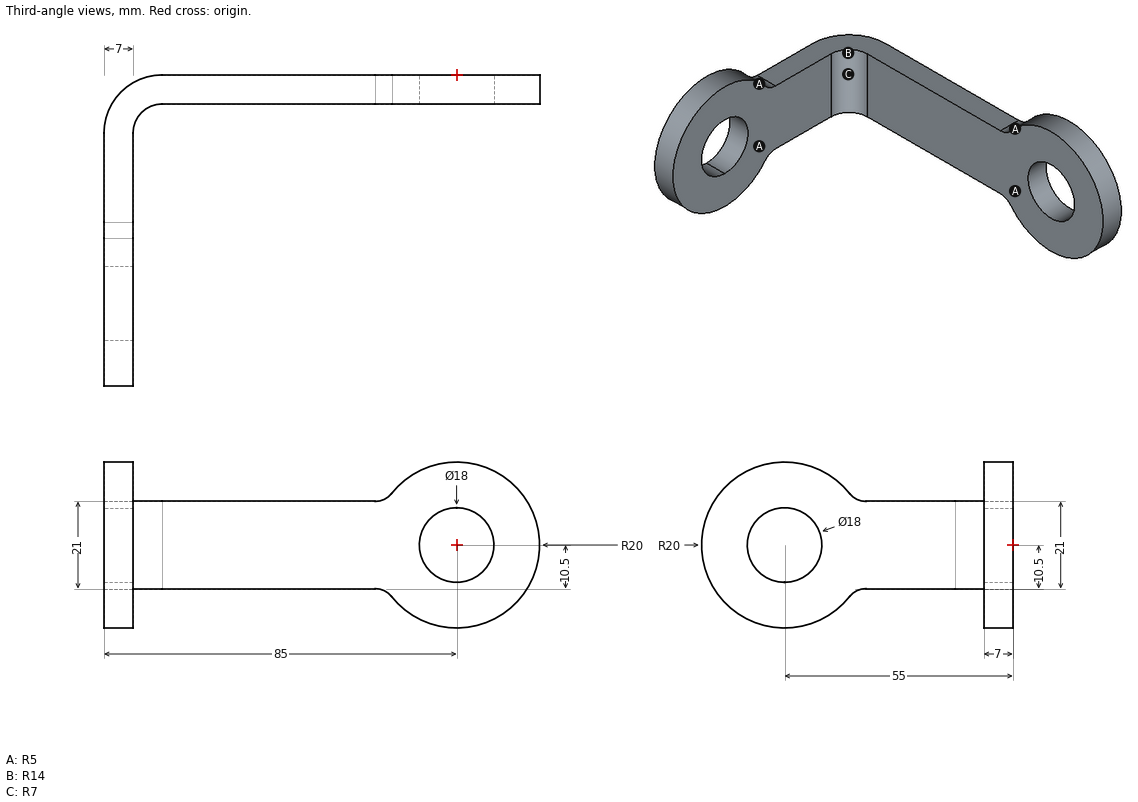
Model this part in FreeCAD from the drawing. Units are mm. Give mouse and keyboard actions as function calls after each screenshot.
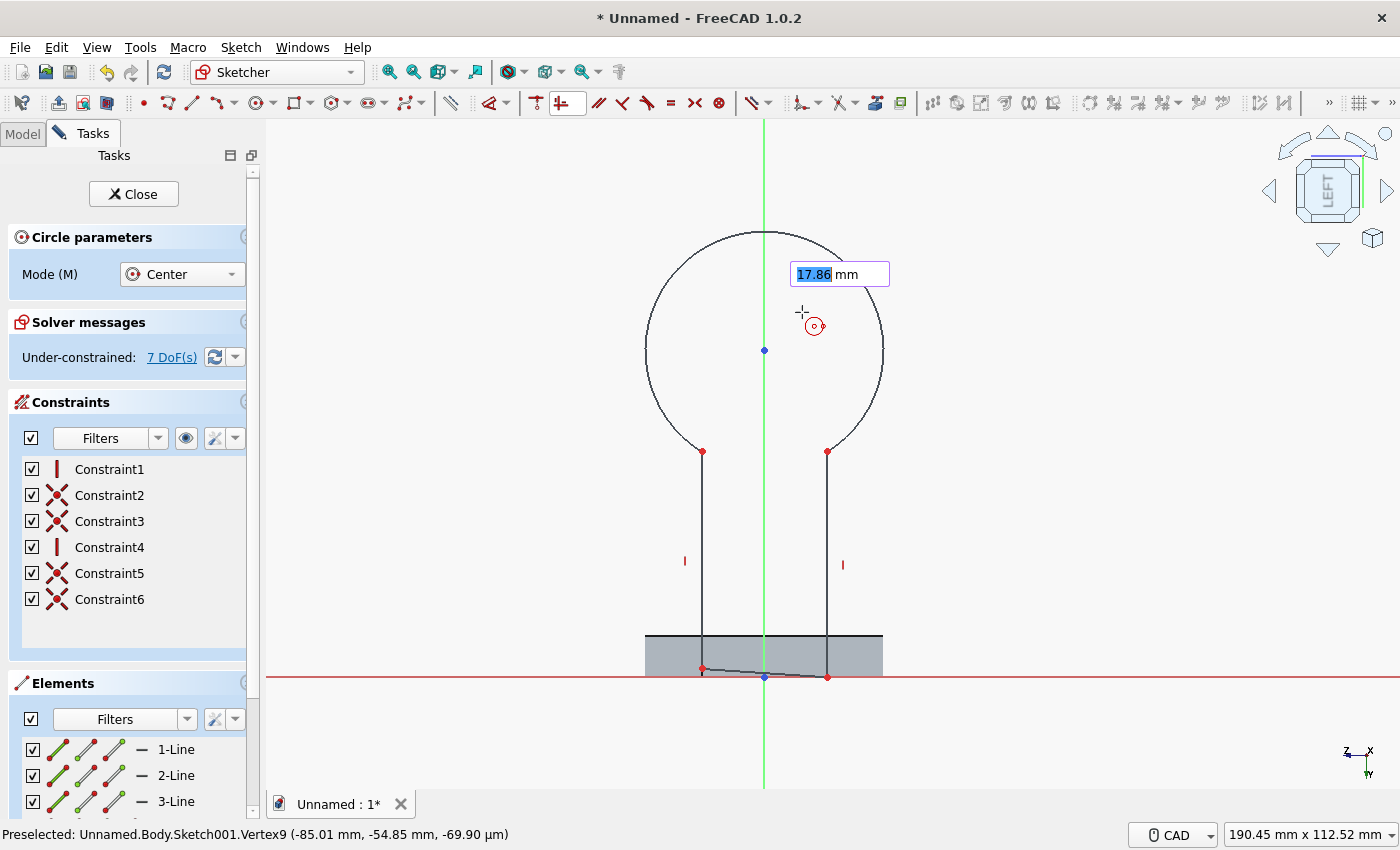
text(18)
key(Return)
key(Escape)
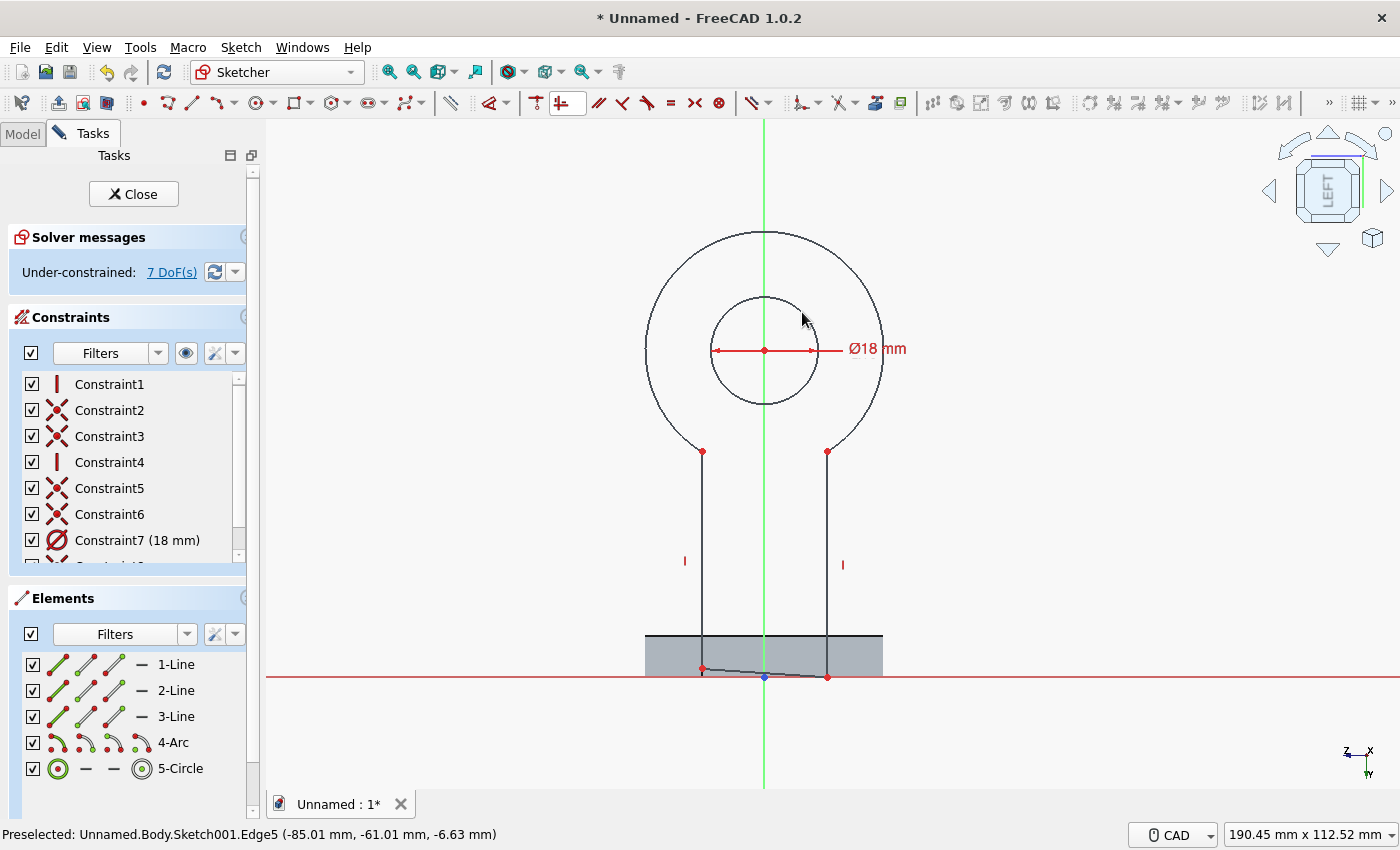
click(789, 675)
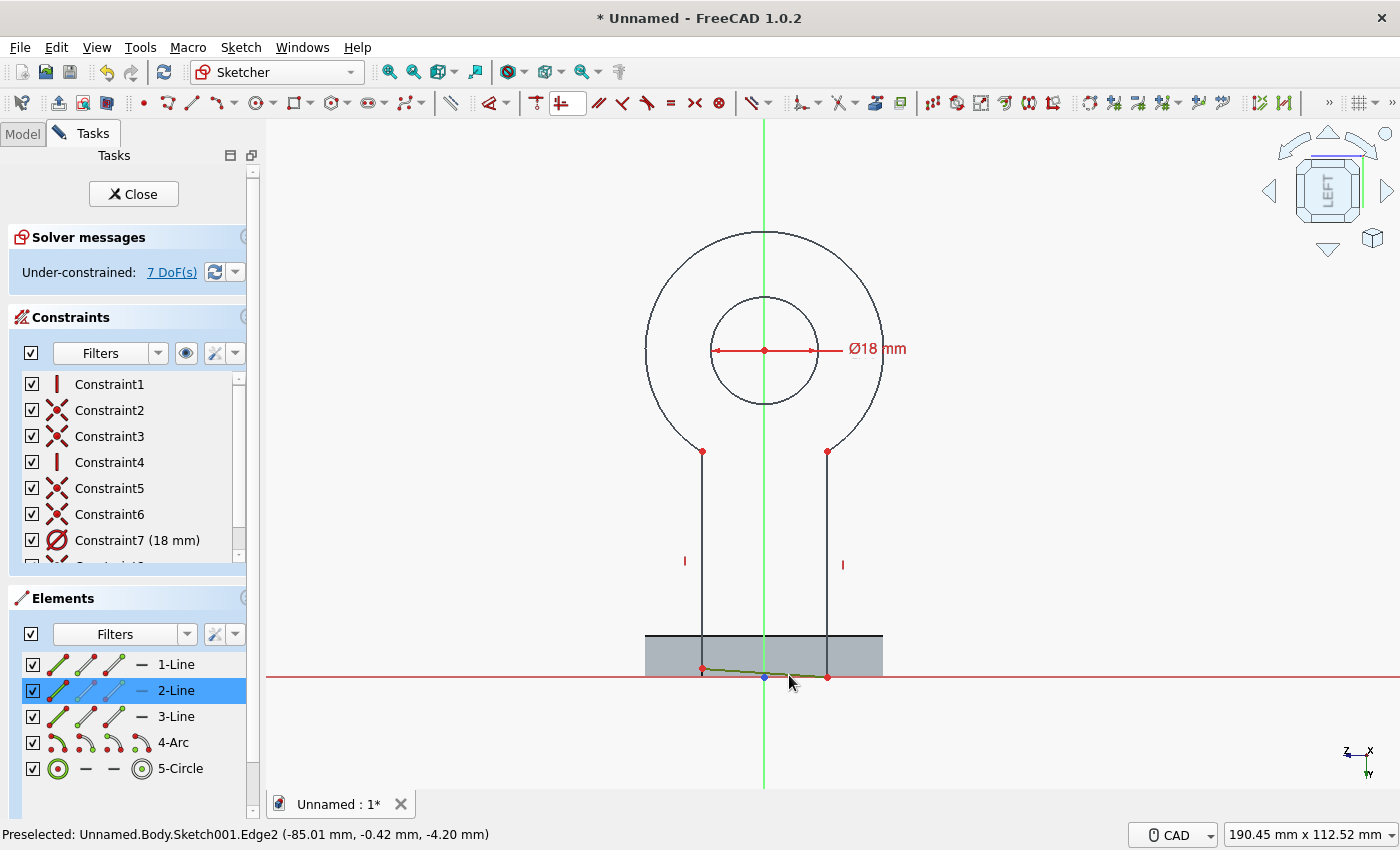
key(h)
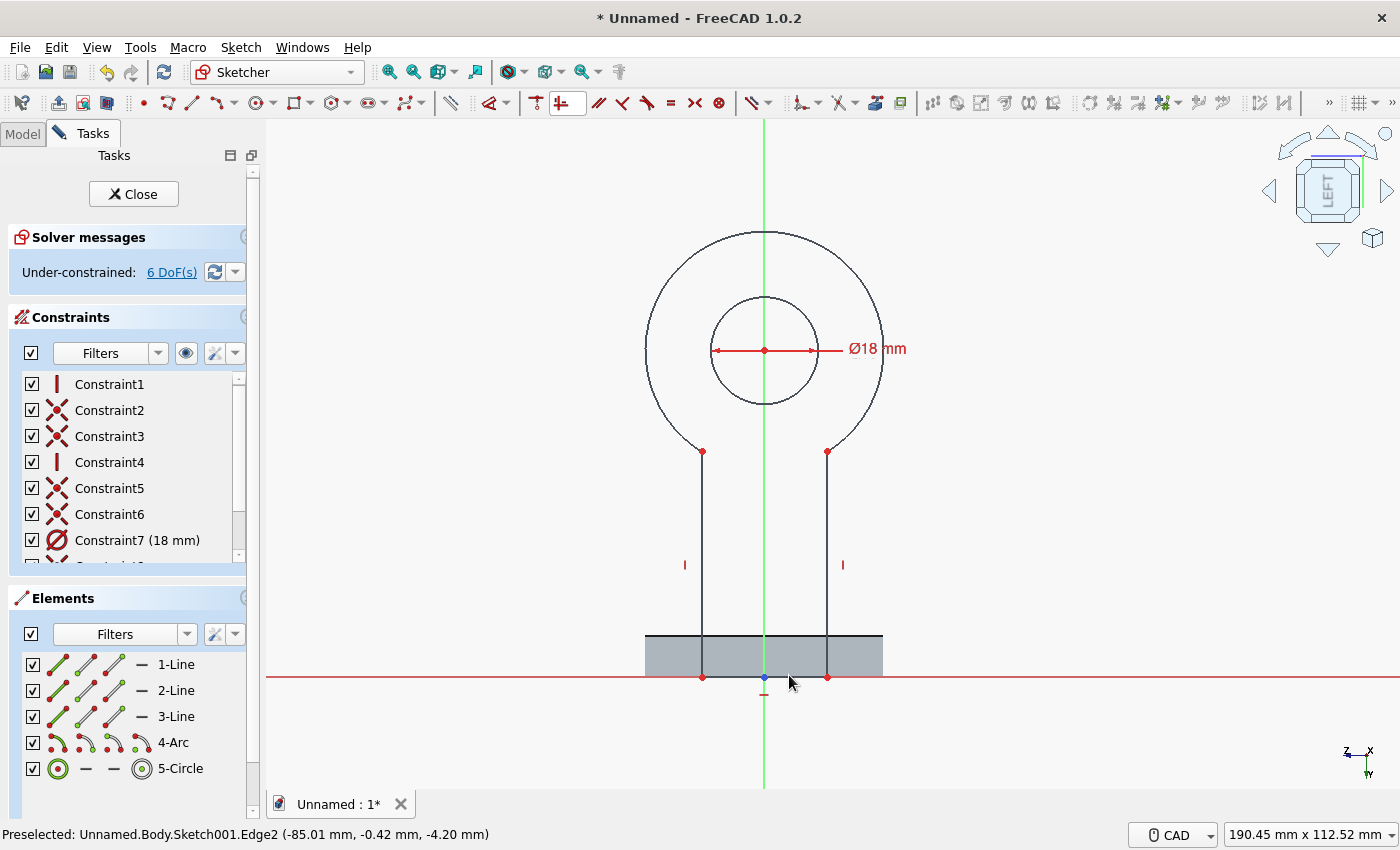
click(765, 351)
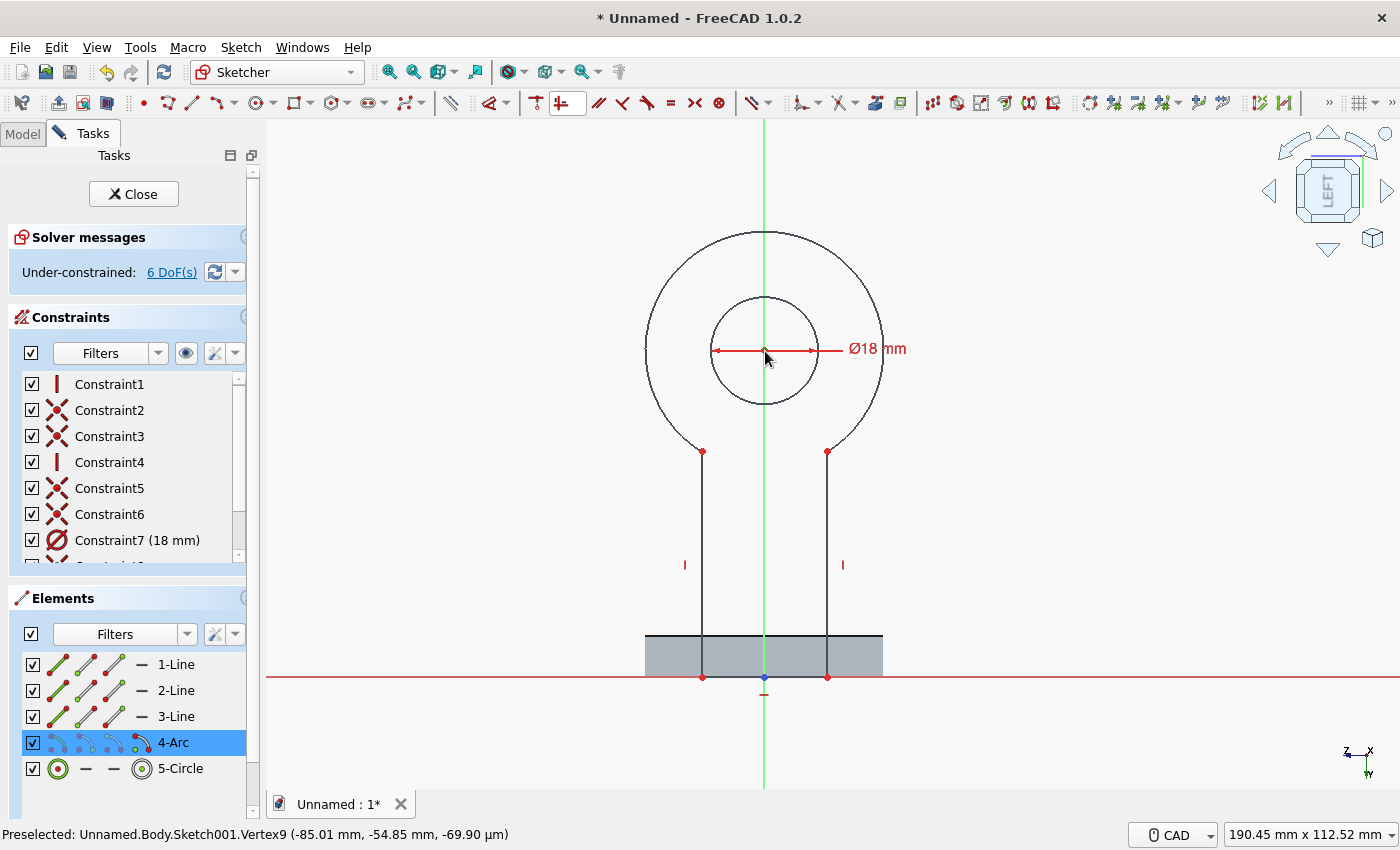
click(764, 717)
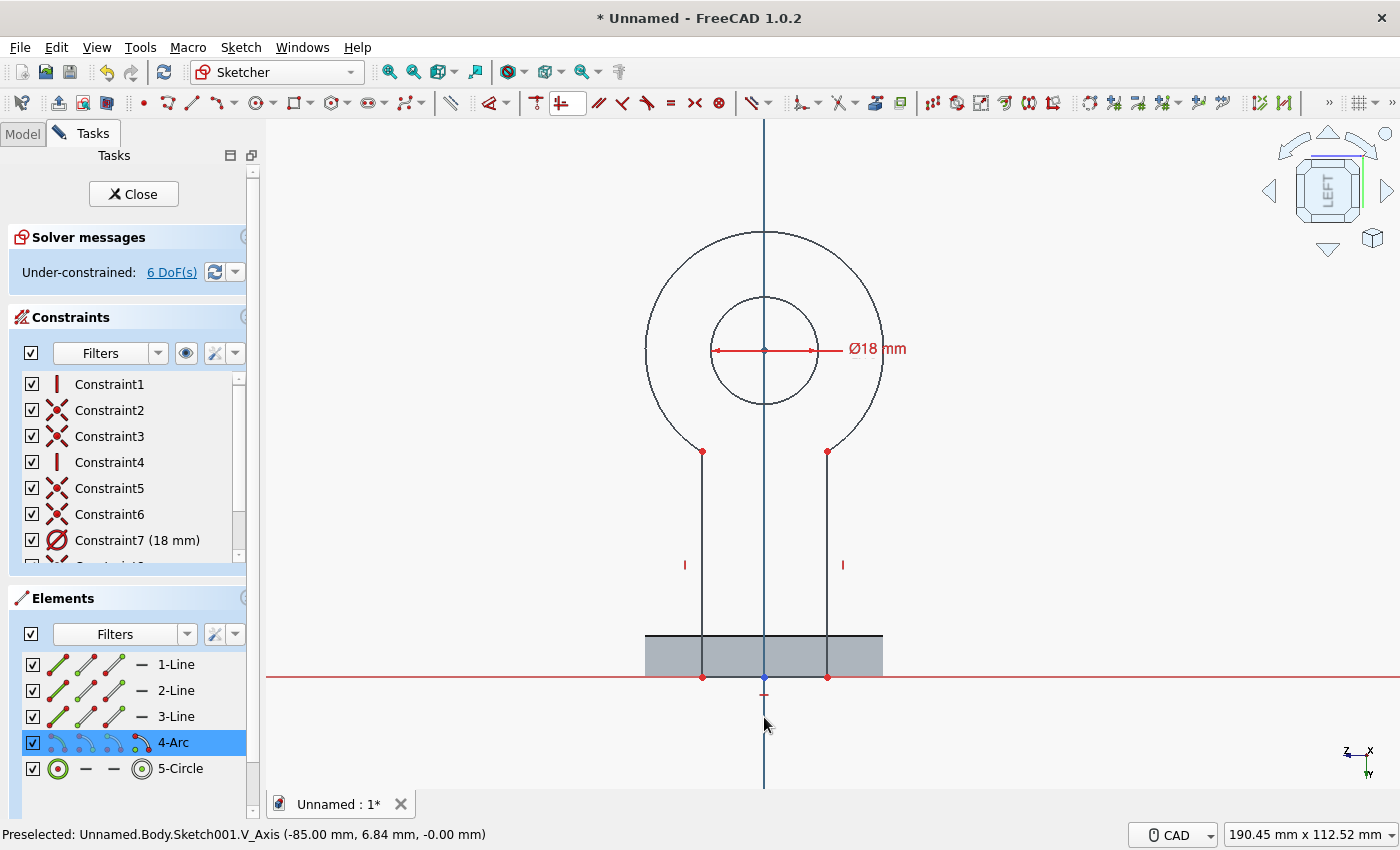
click(536, 104)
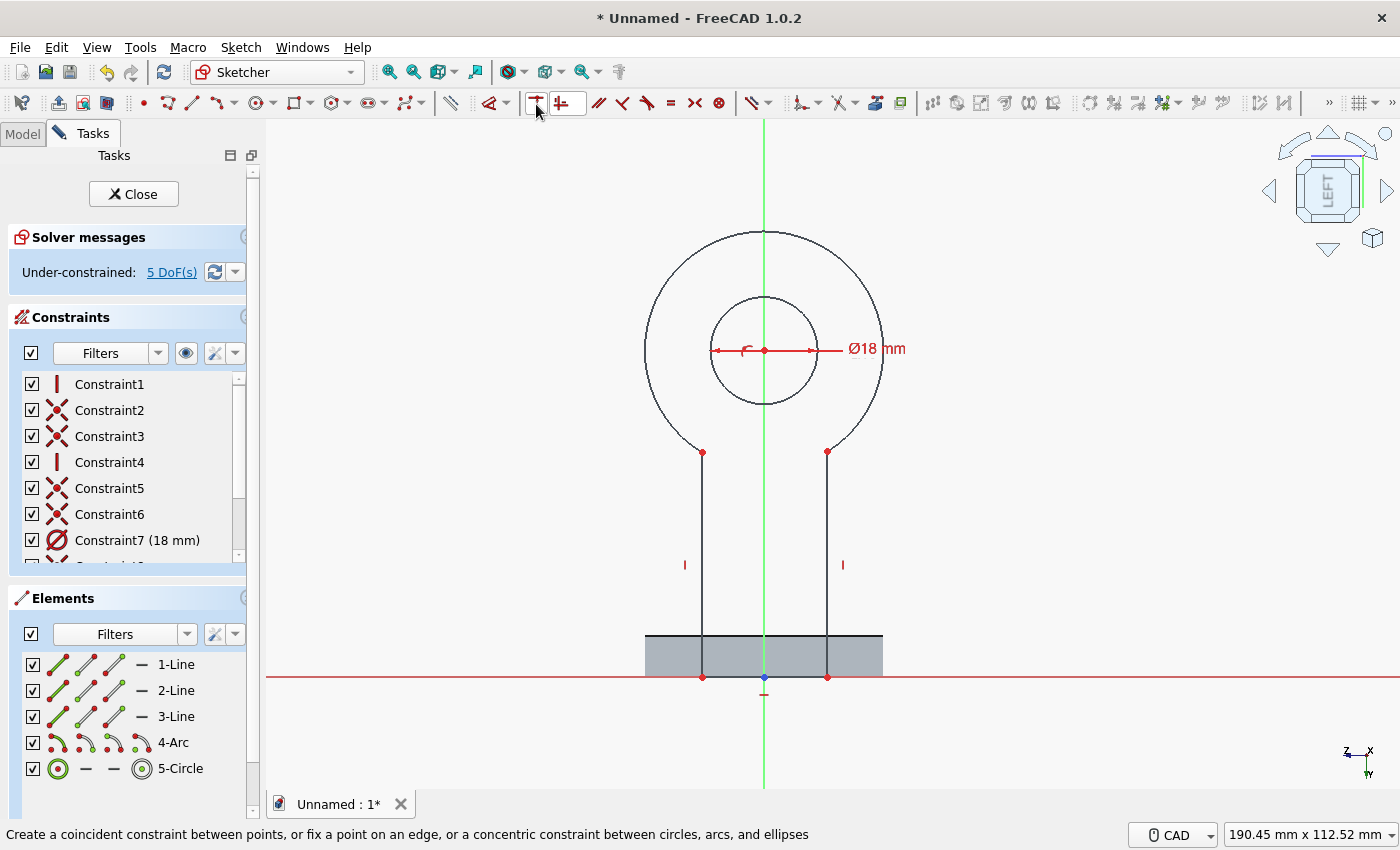
click(490, 104)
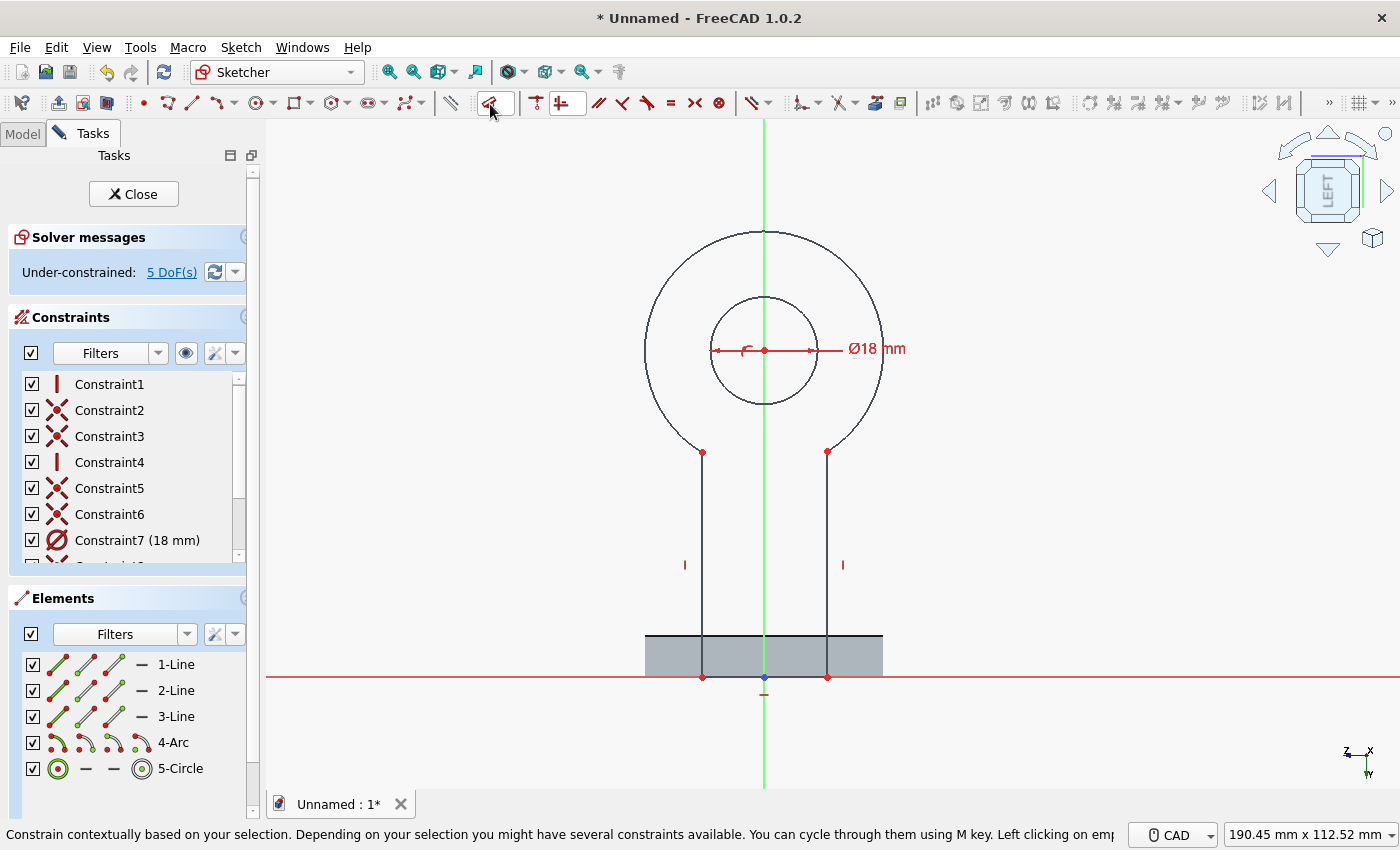
click(866, 289)
click(893, 272)